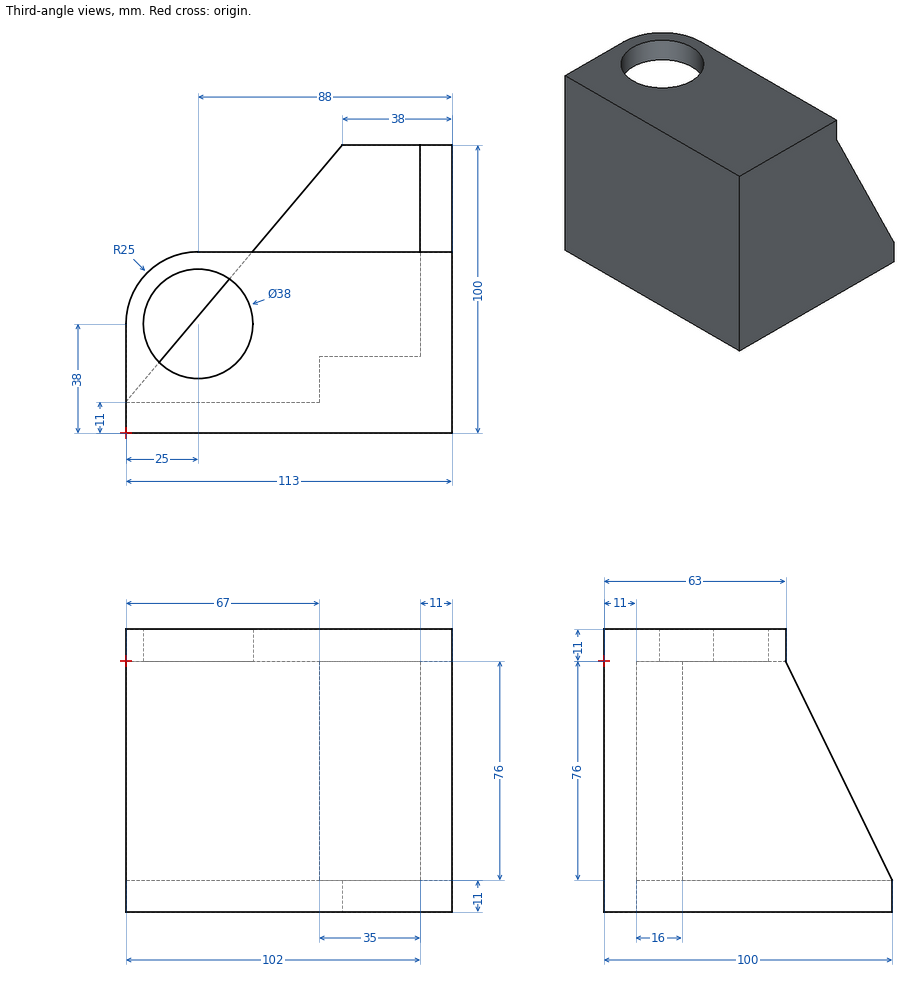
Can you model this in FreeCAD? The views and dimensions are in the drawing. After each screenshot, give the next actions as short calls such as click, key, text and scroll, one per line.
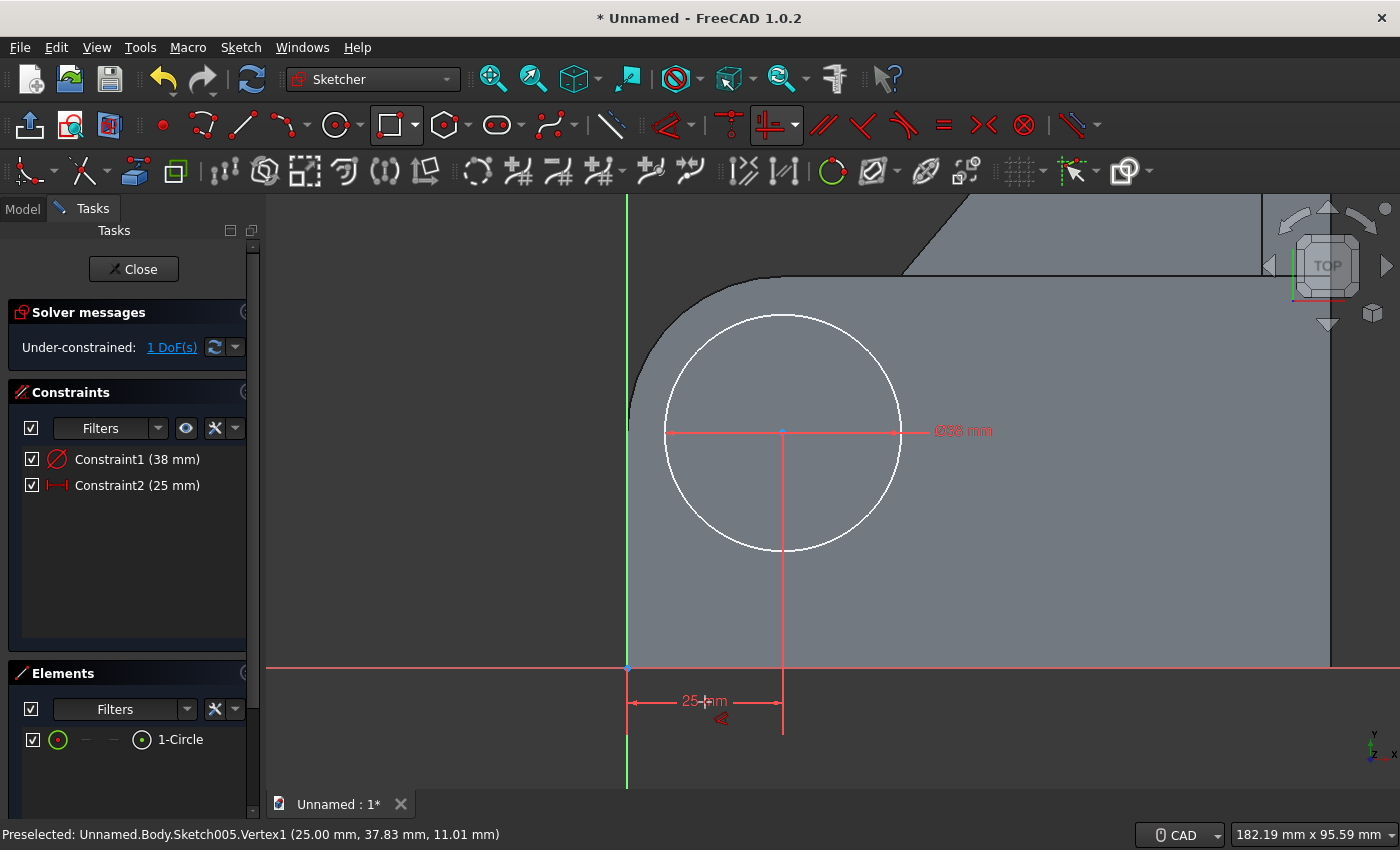
click(783, 433)
click(593, 551)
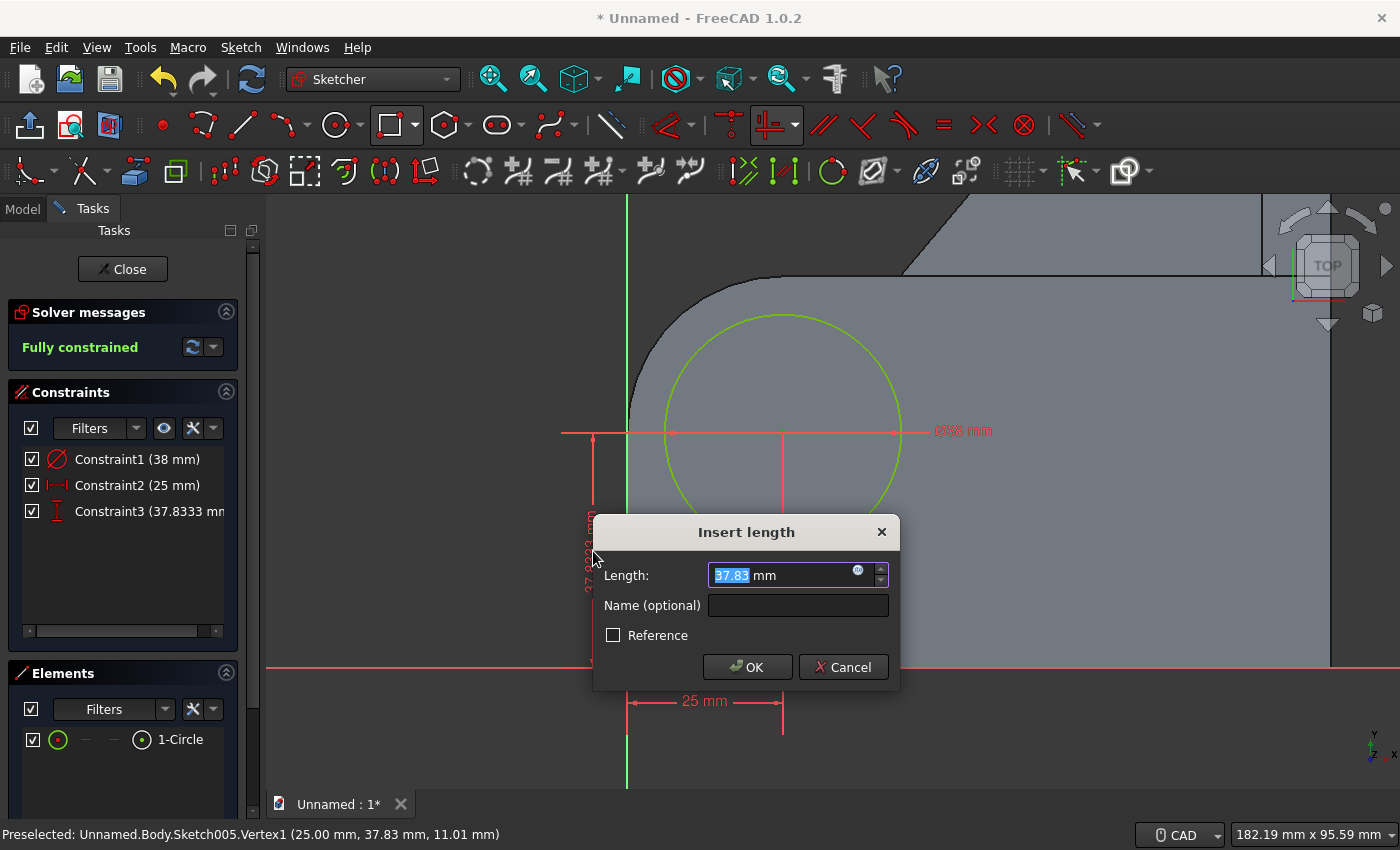
text(38)
key(Return)
key(Escape)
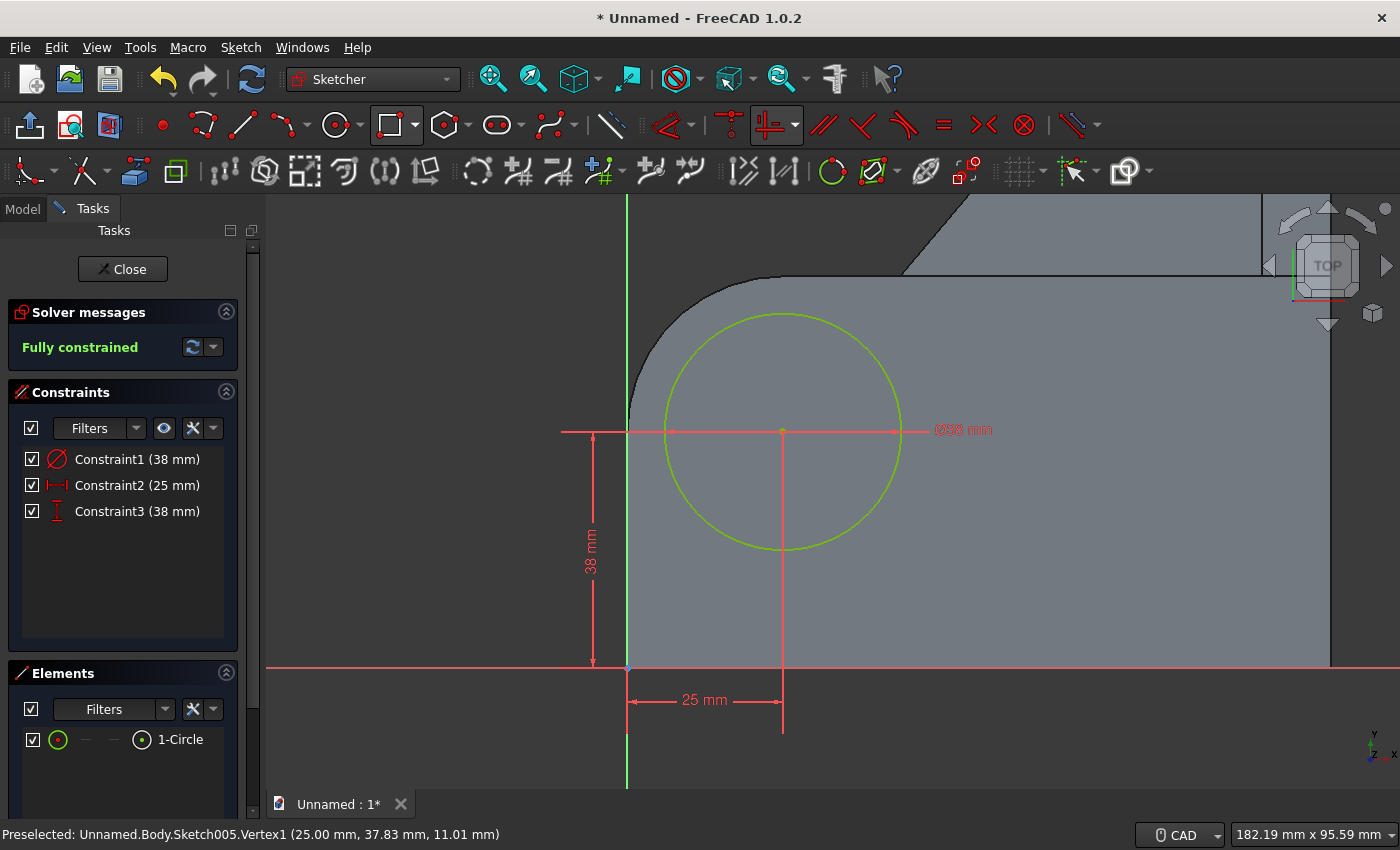
click(123, 269)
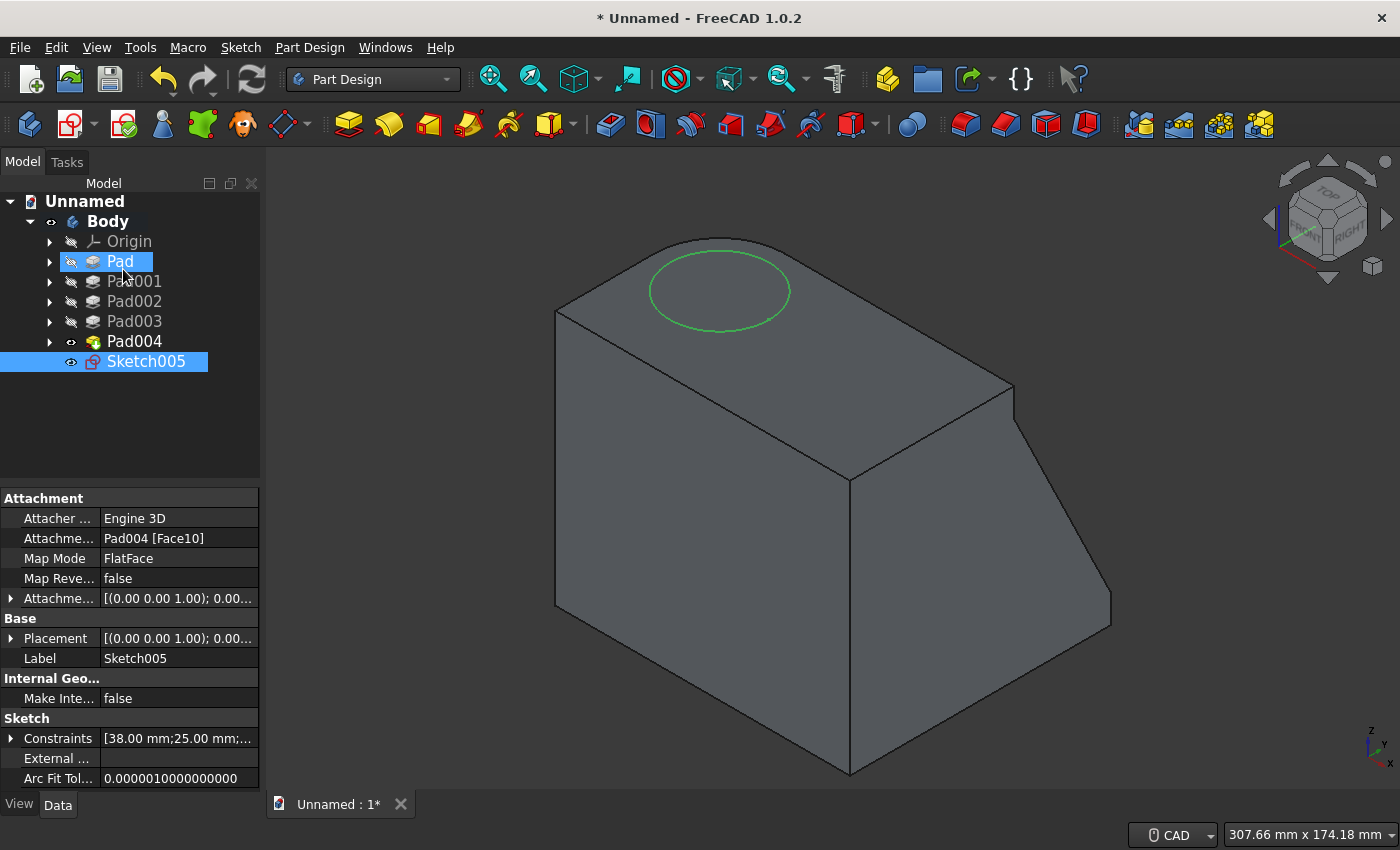
click(612, 124)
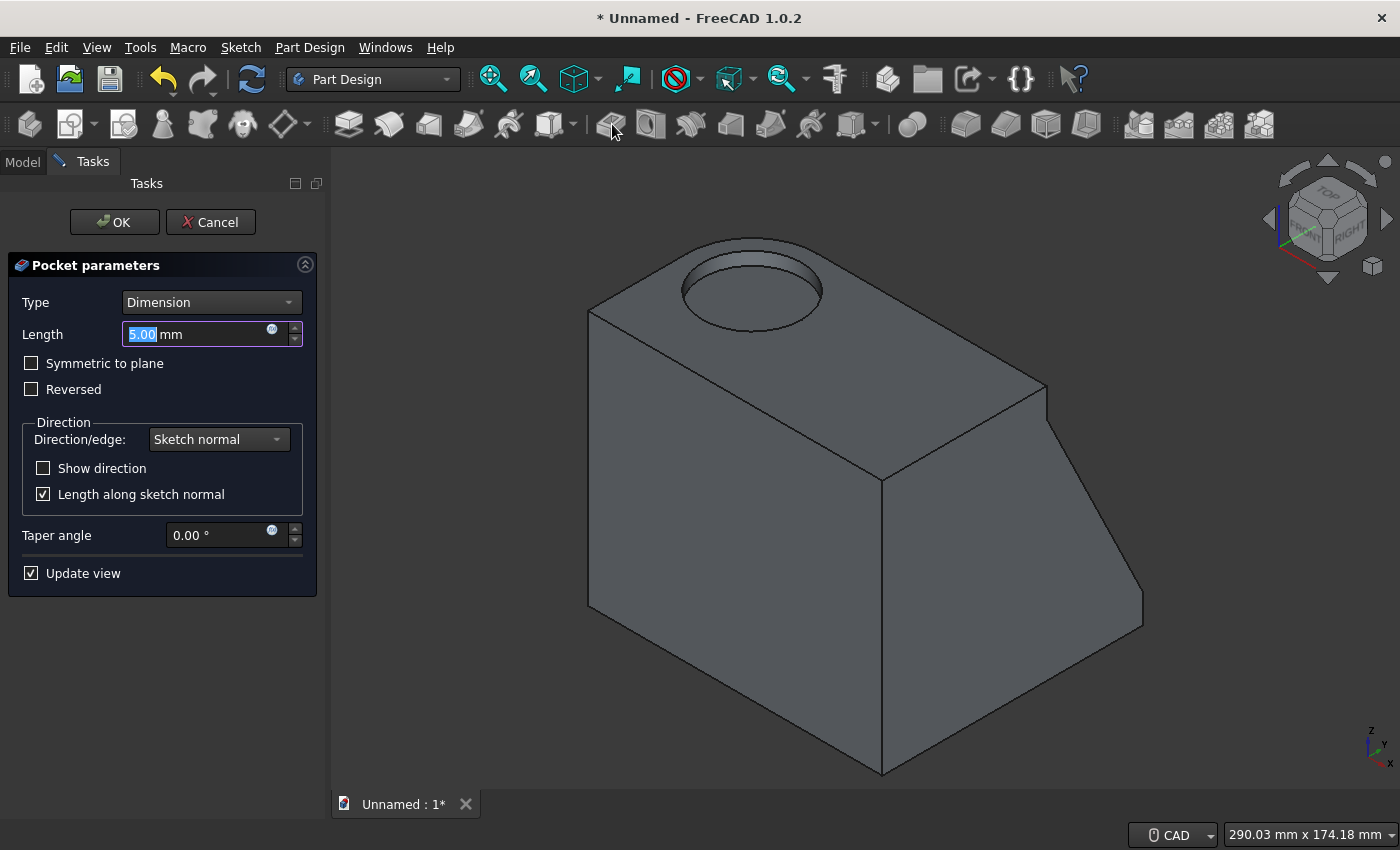
text(11)
key(Tab)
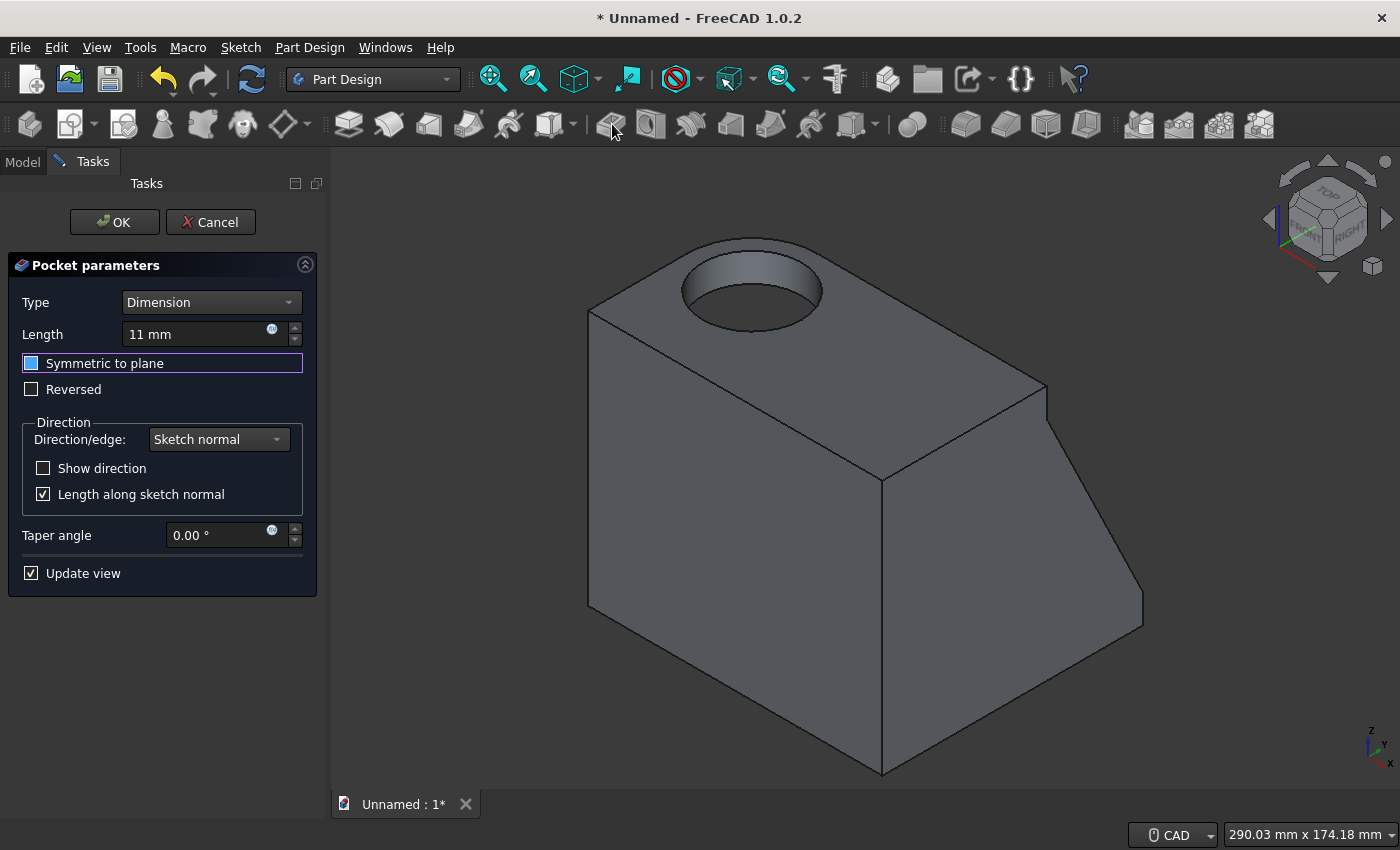
click(115, 222)